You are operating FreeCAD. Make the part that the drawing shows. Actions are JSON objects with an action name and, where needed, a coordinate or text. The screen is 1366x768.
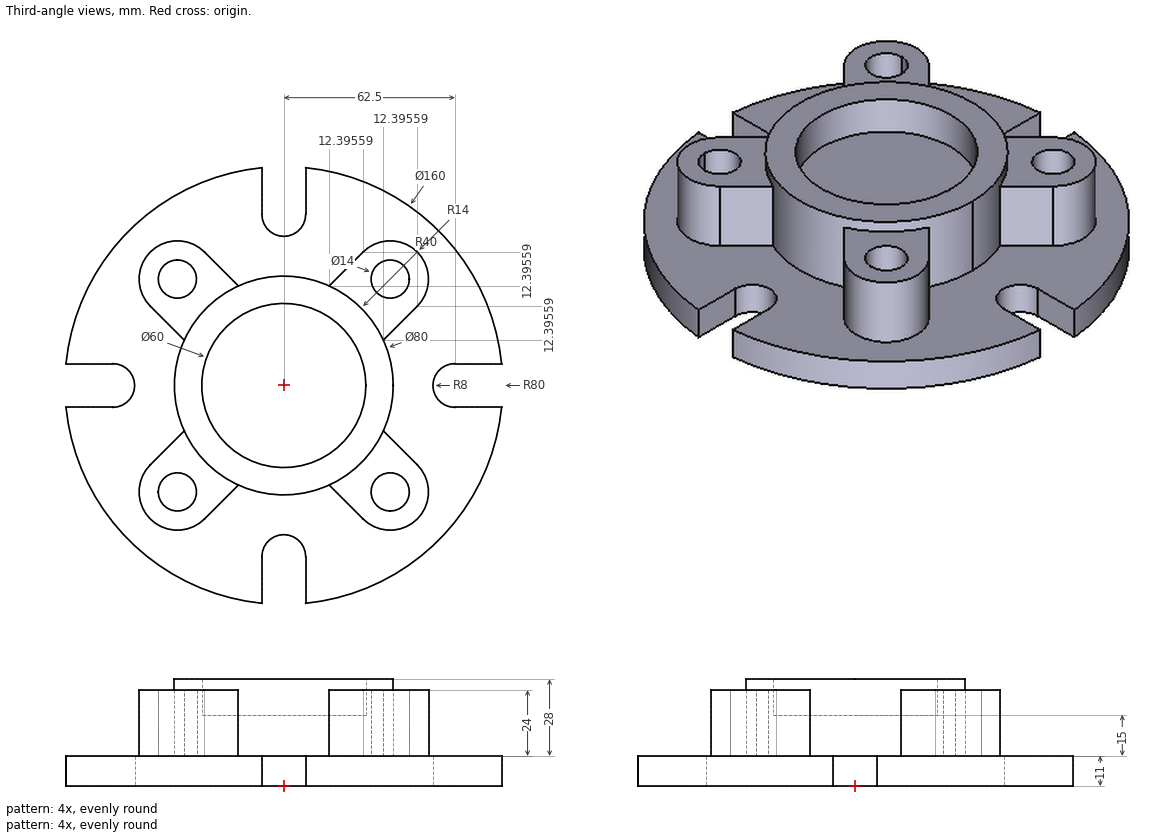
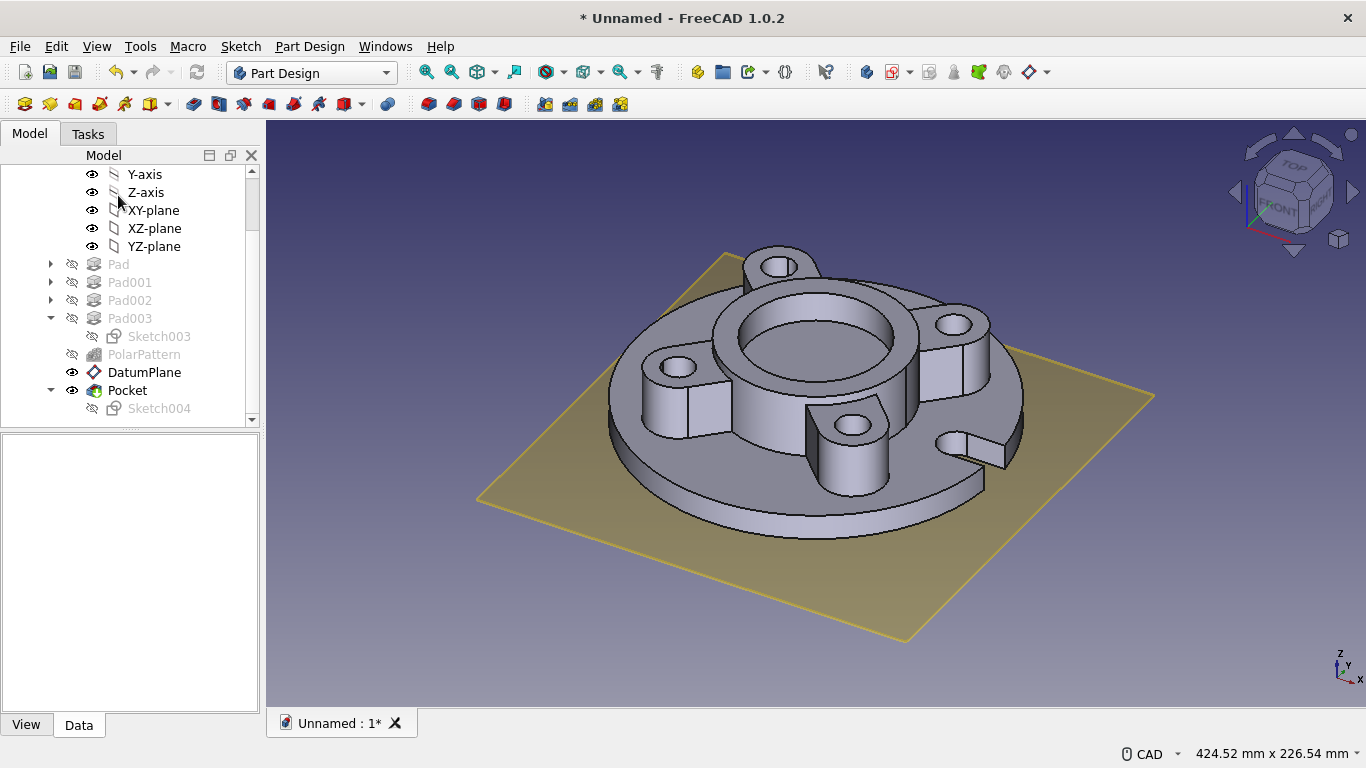
{"action": "left_click", "coordinate": [117, 372]}
{"action": "key", "text": "space"}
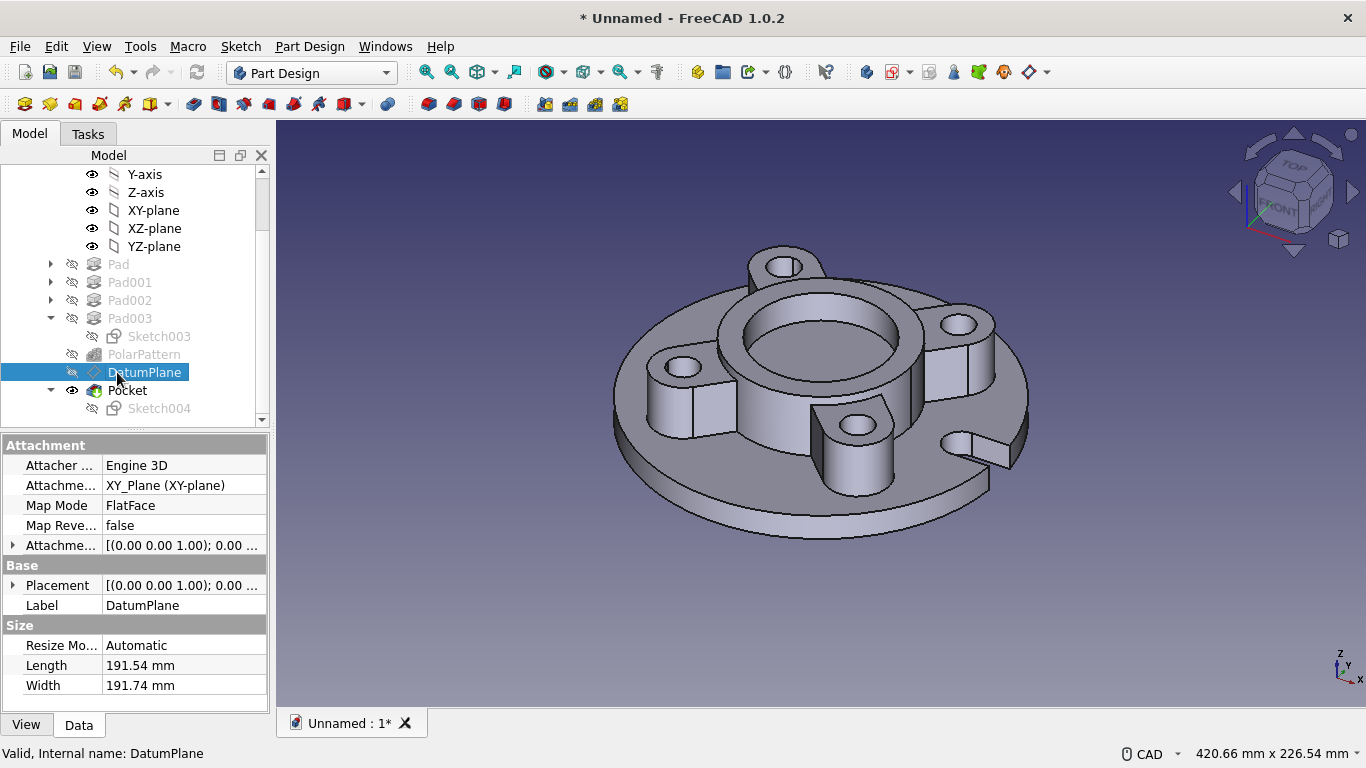
{"action": "left_click", "coordinate": [117, 390]}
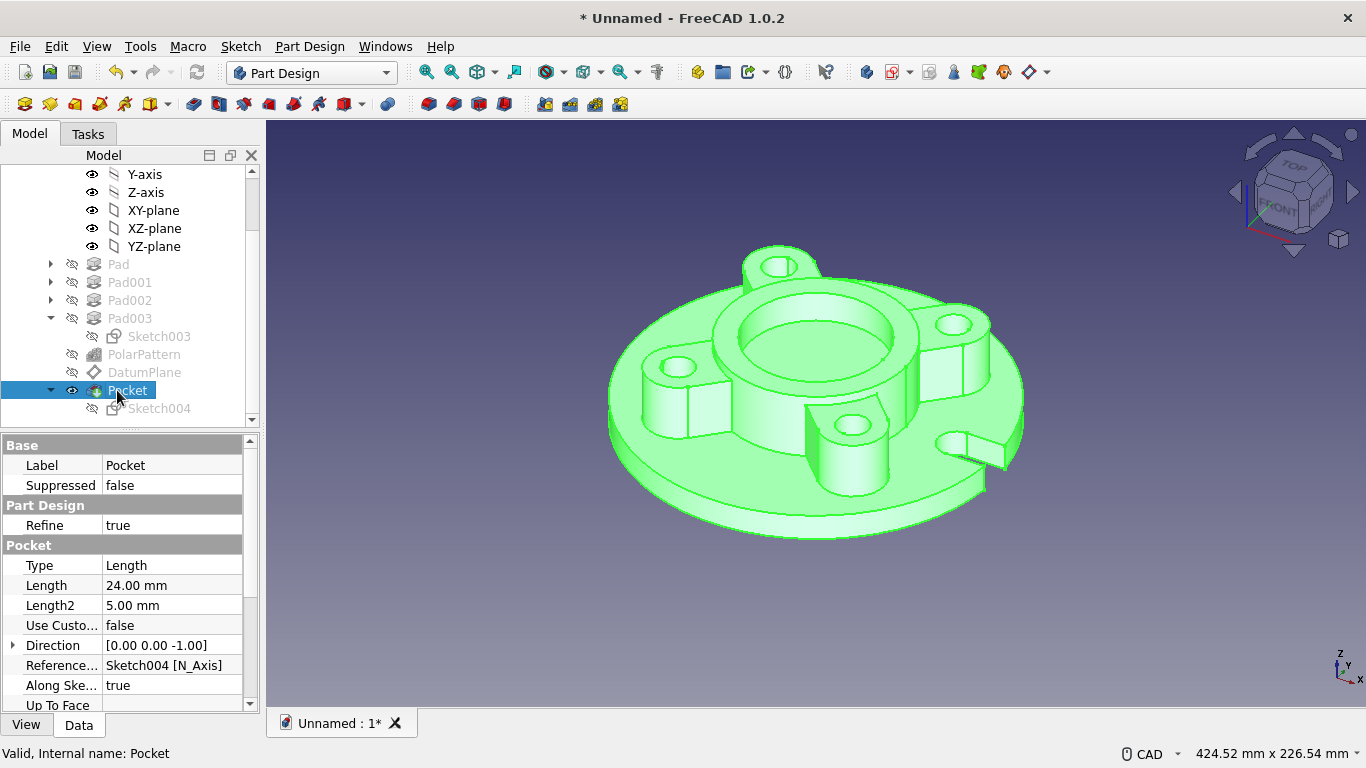
{"action": "left_click", "coordinate": [595, 104]}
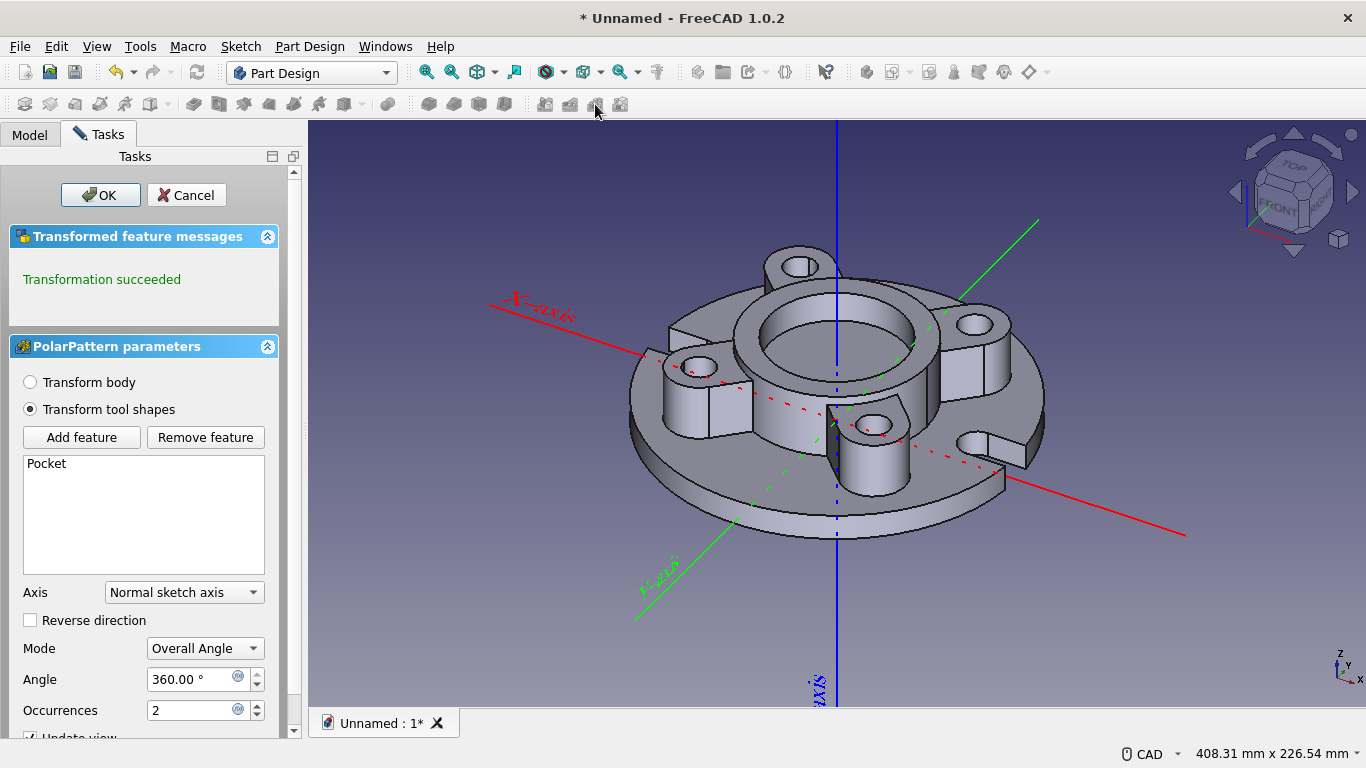
{"action": "left_click", "coordinate": [185, 592]}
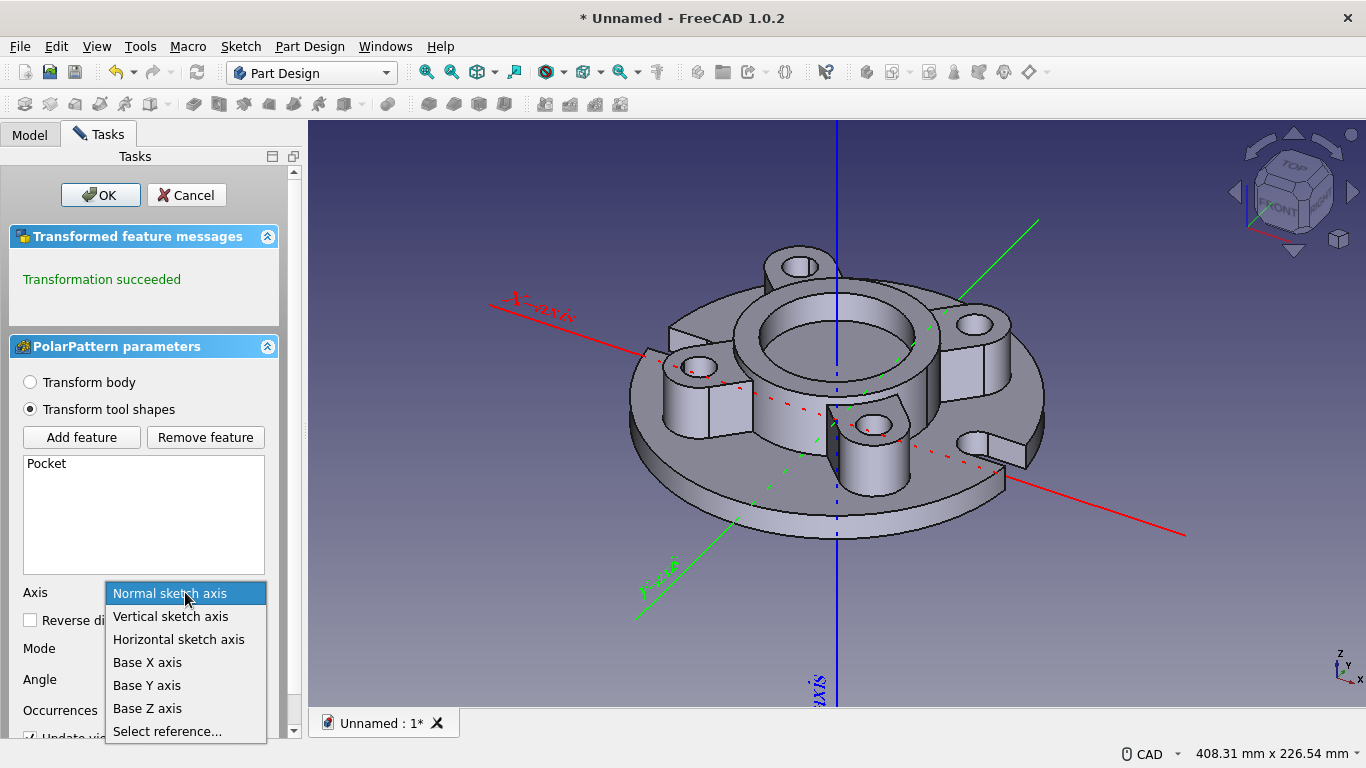
{"action": "left_click", "coordinate": [184, 708]}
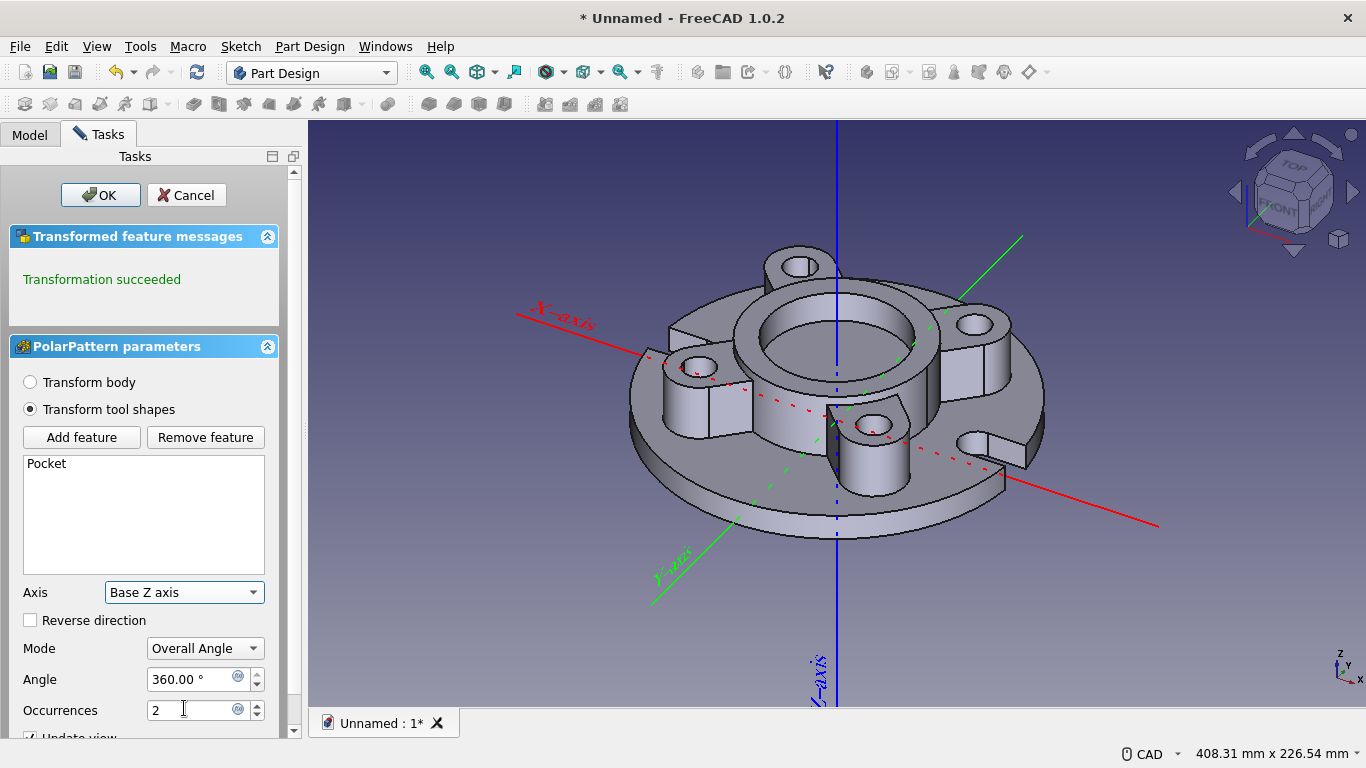
{"action": "triple_click", "coordinate": [199, 710]}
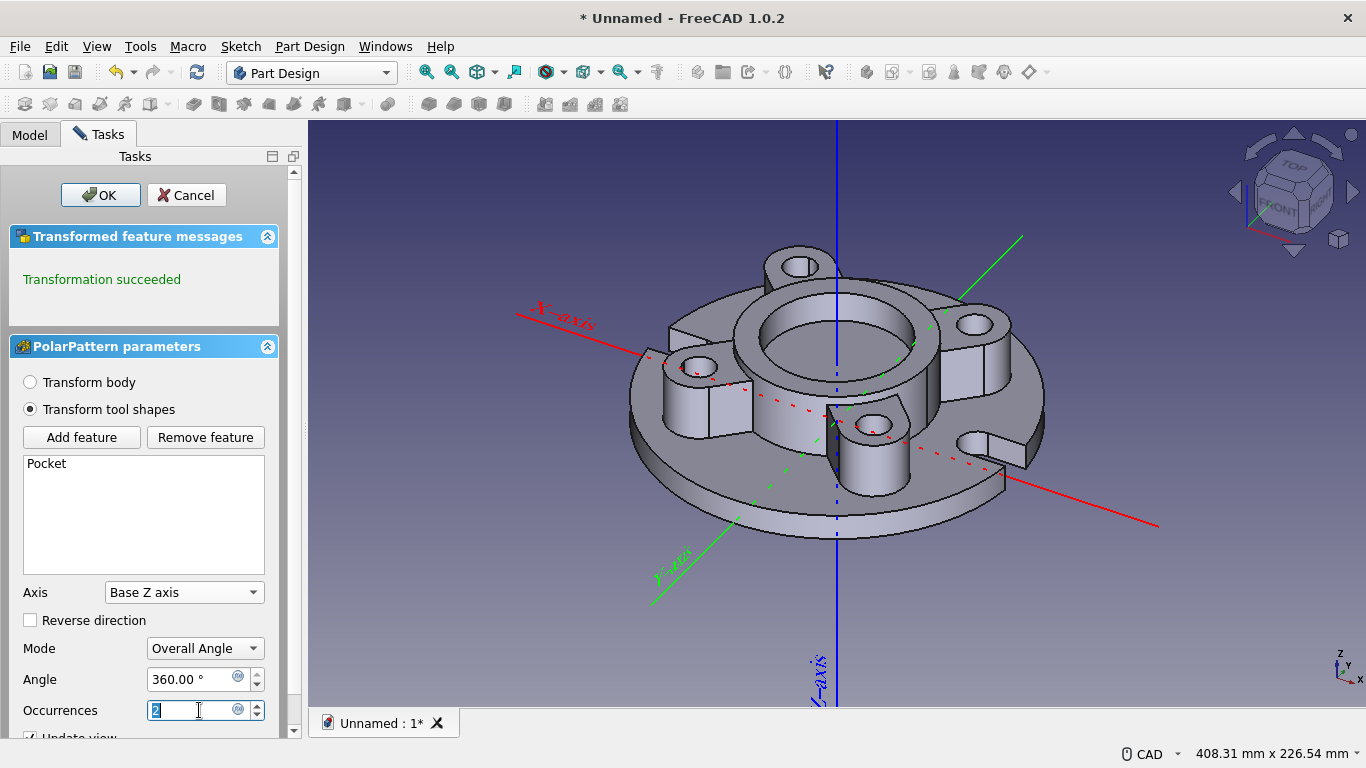
{"action": "type", "text": "4"}
{"action": "key", "text": "Tab"}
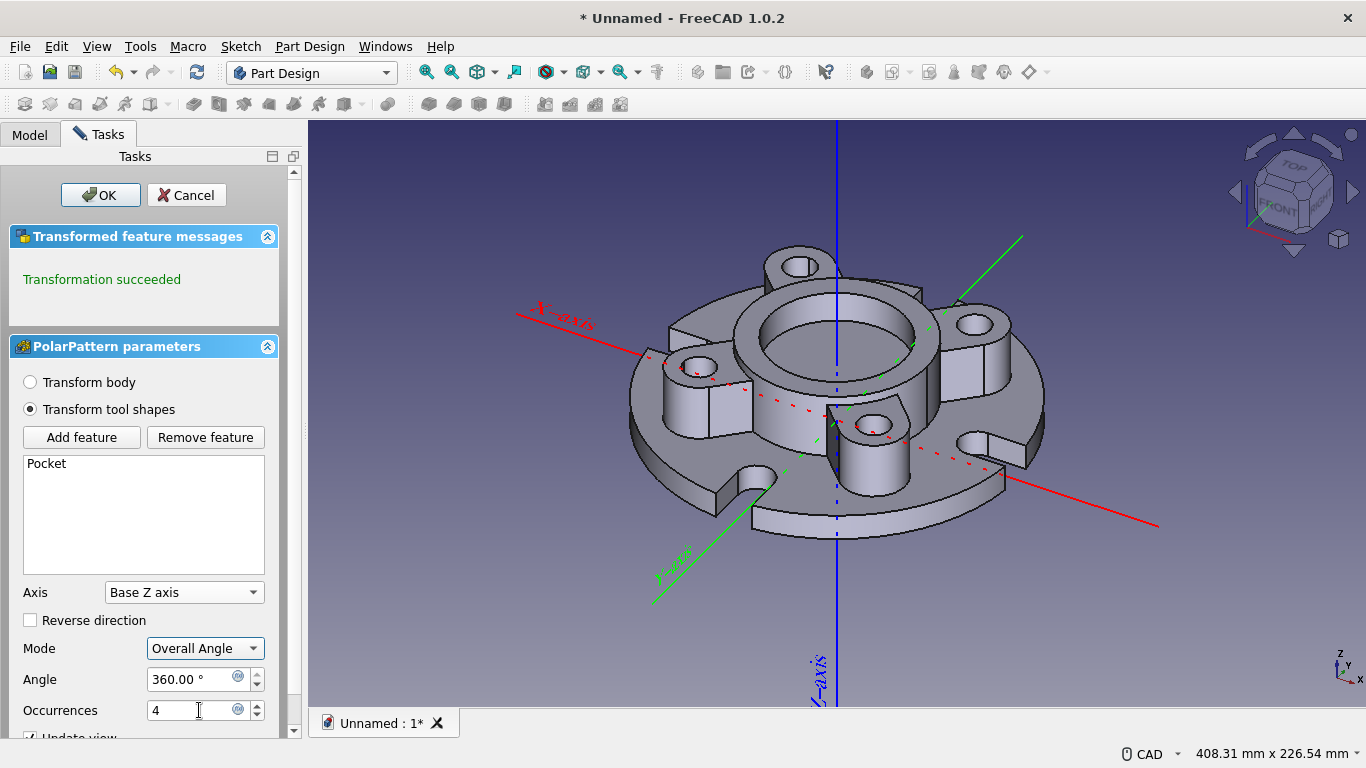
{"action": "left_click", "coordinate": [101, 195]}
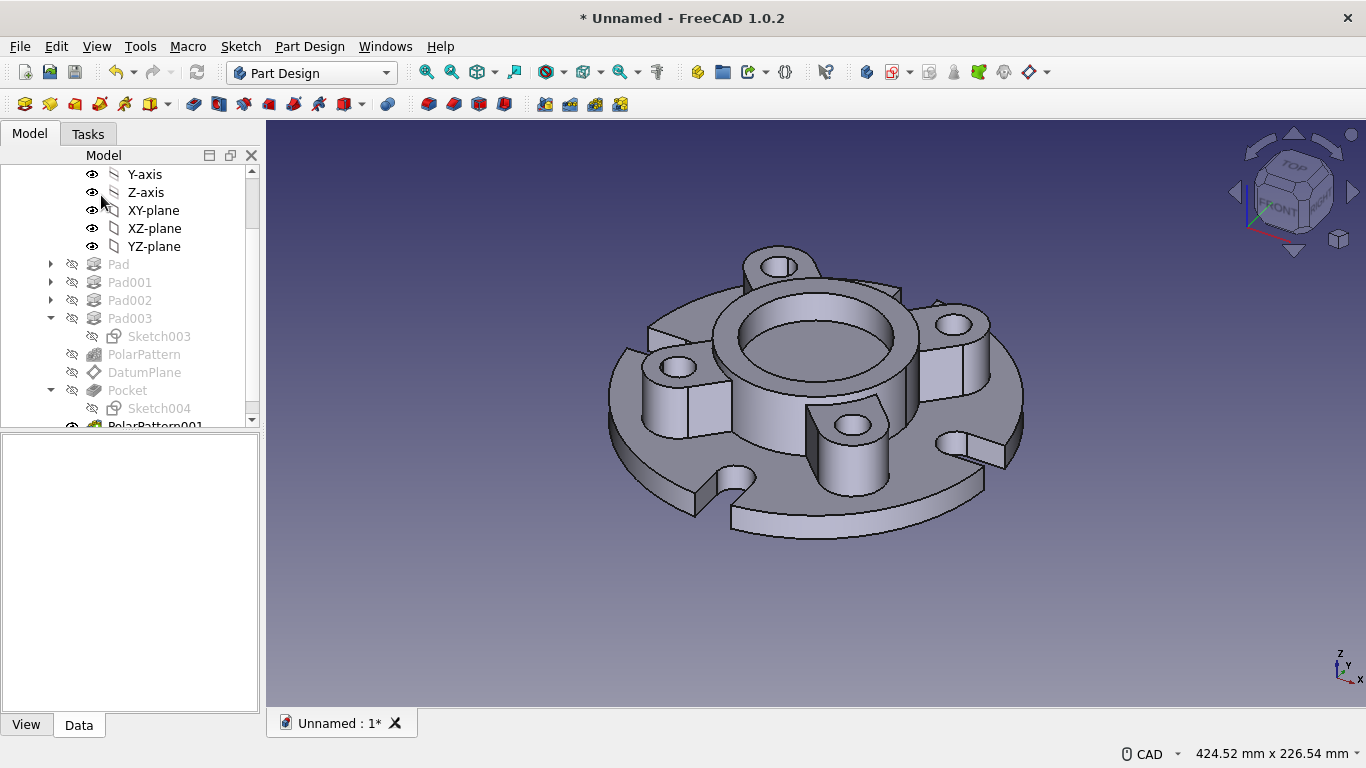
{"action": "key", "text": "0"}